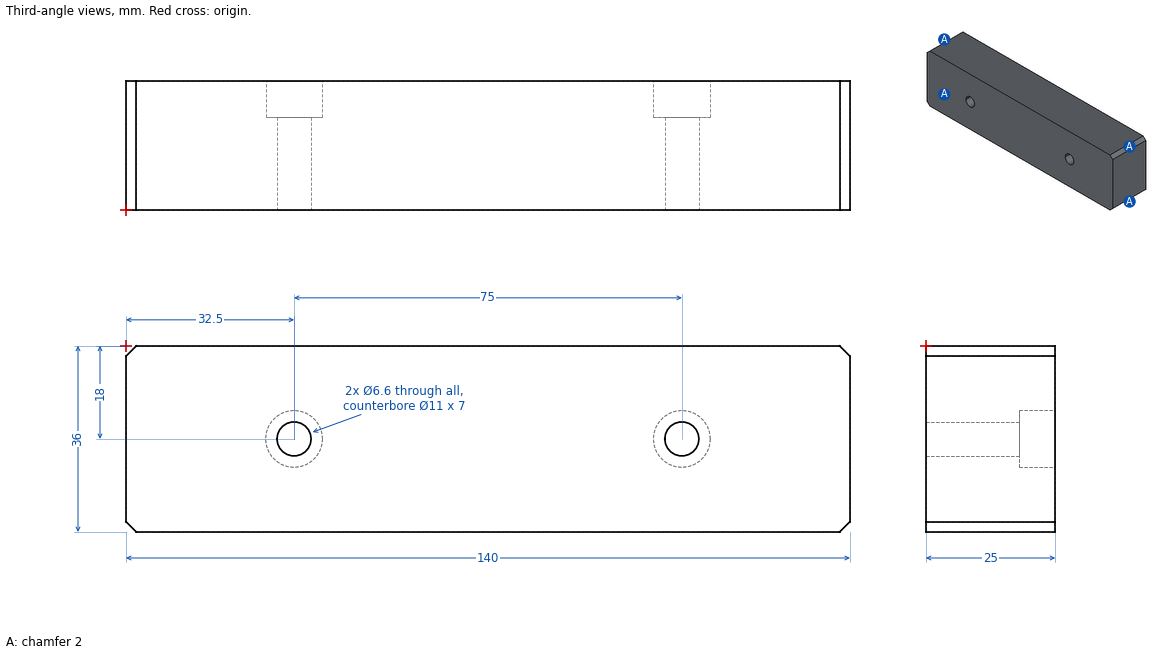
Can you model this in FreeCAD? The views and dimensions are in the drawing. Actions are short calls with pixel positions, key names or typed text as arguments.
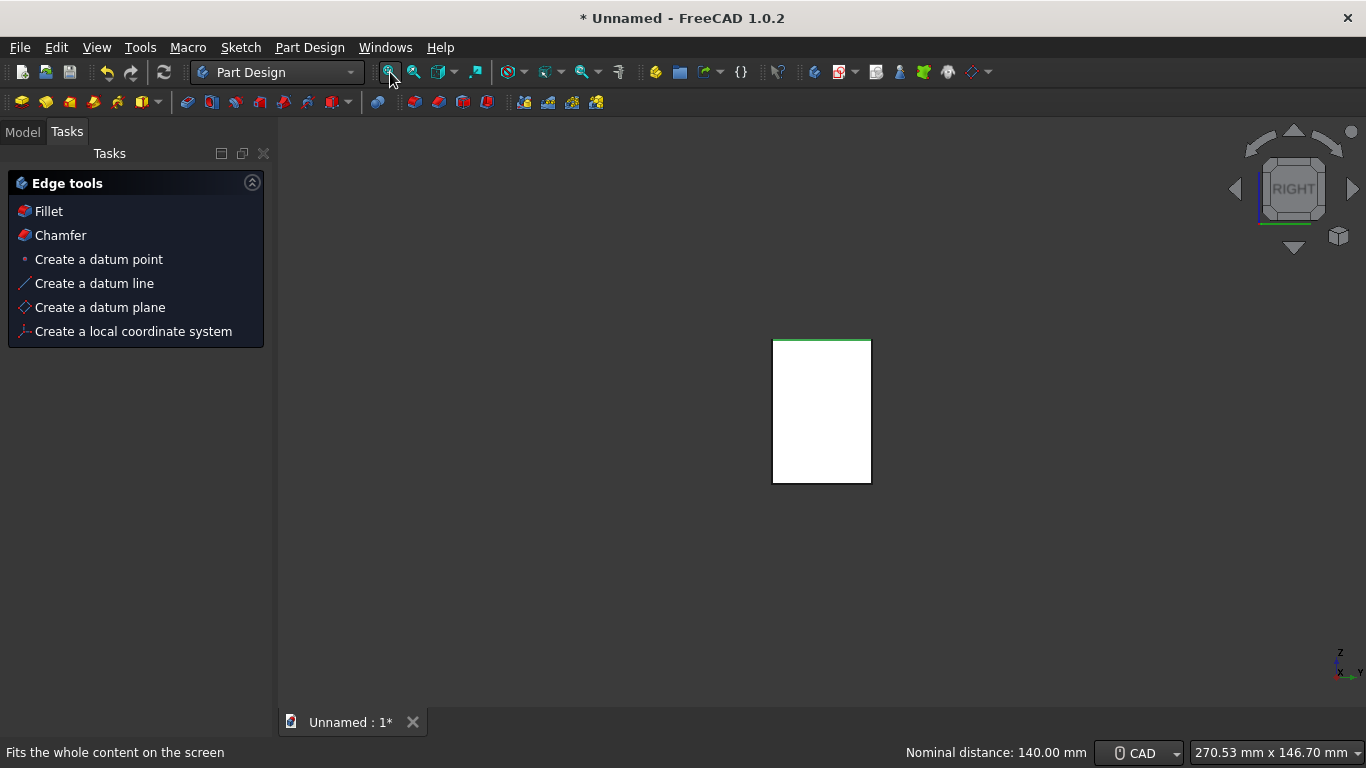
click(822, 483, ctrl)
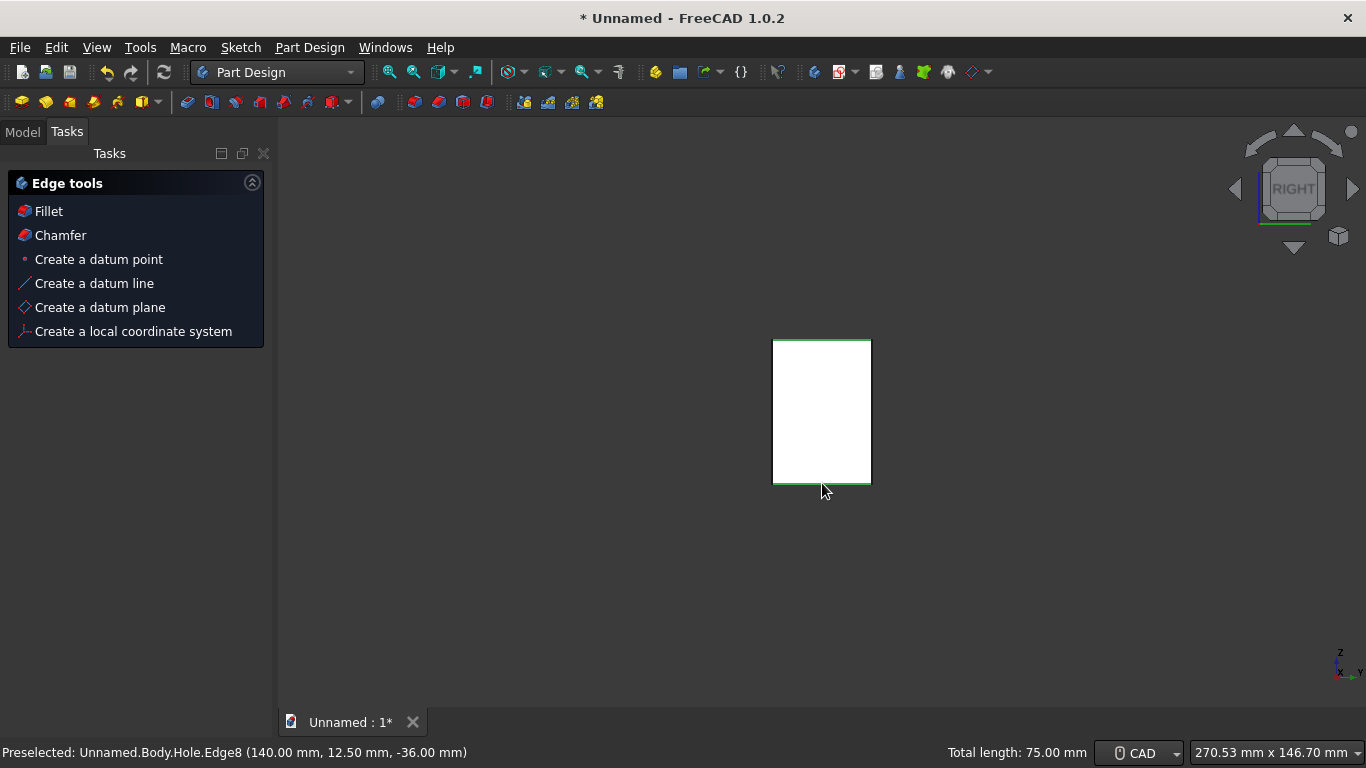
key(5)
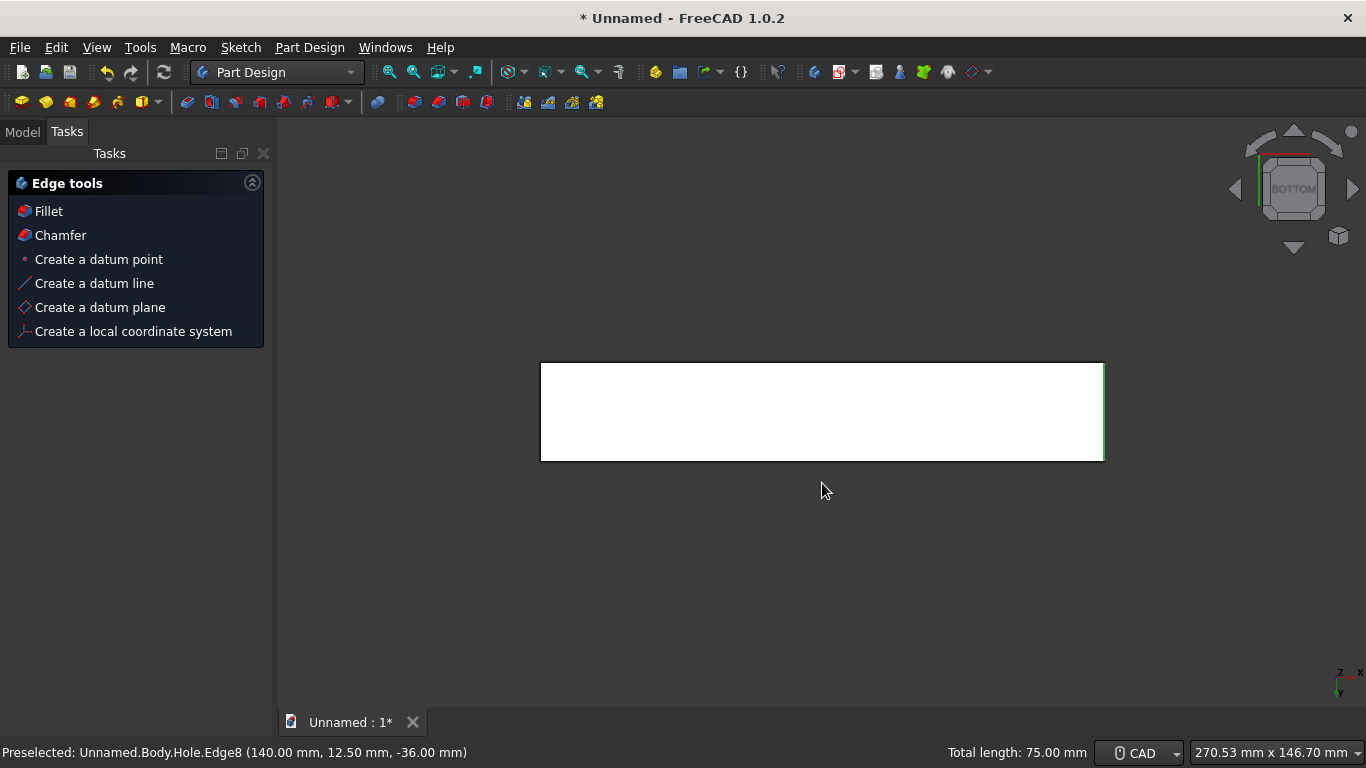
click(540, 411, ctrl)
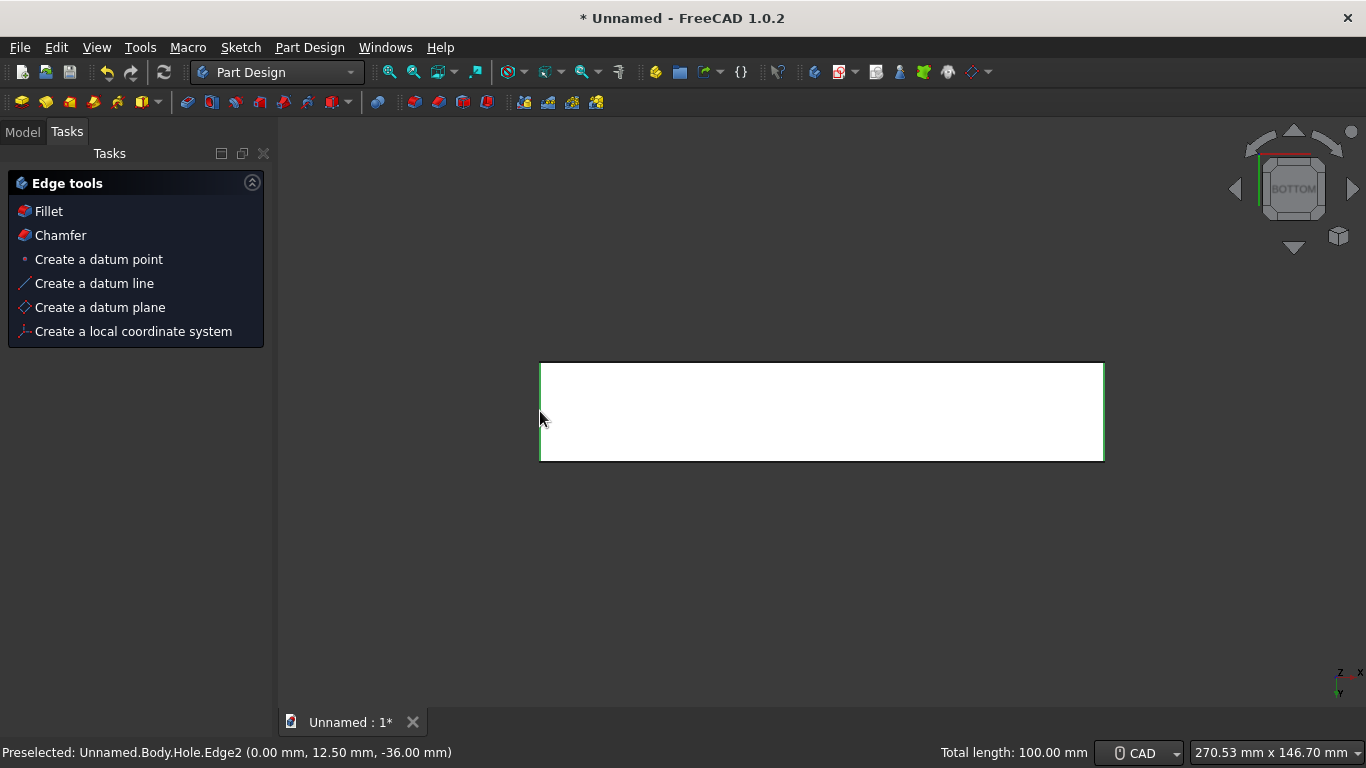
click(440, 102)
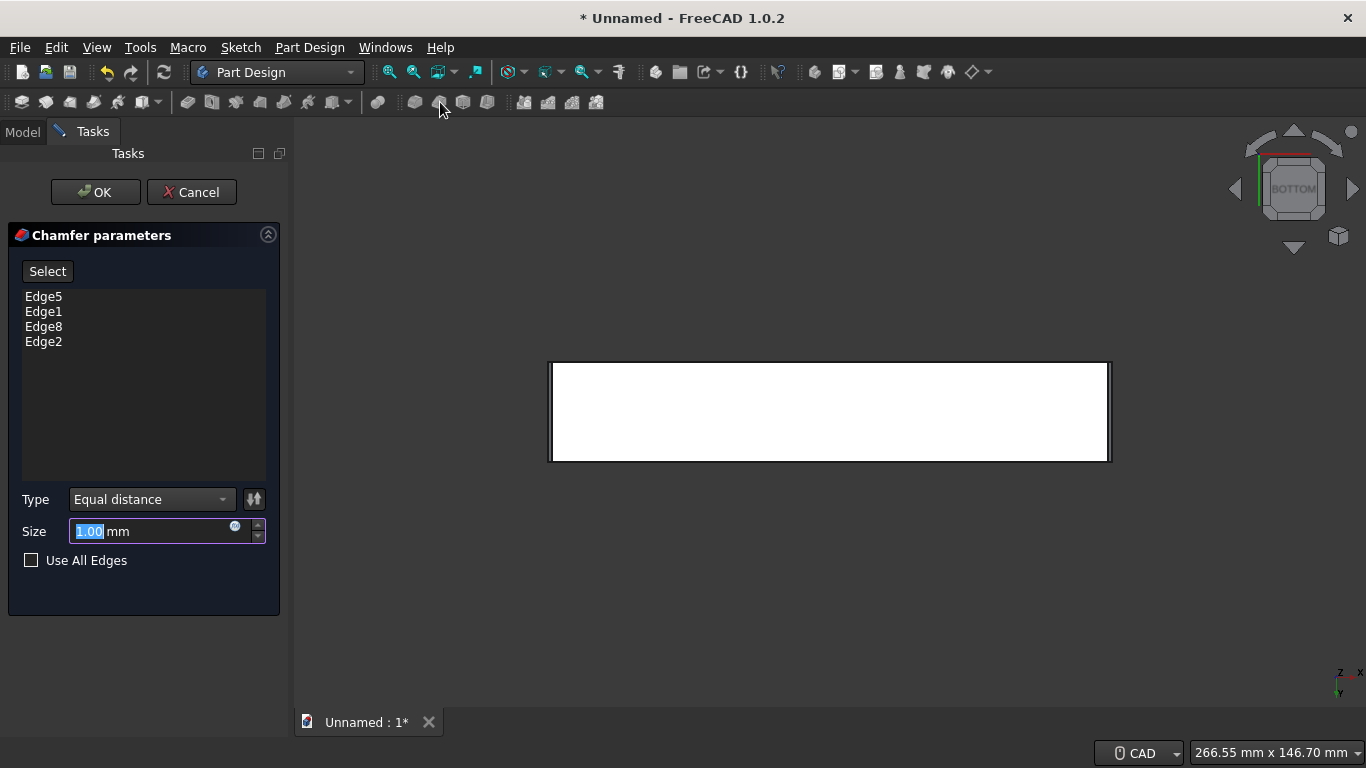
text(2)
key(Tab)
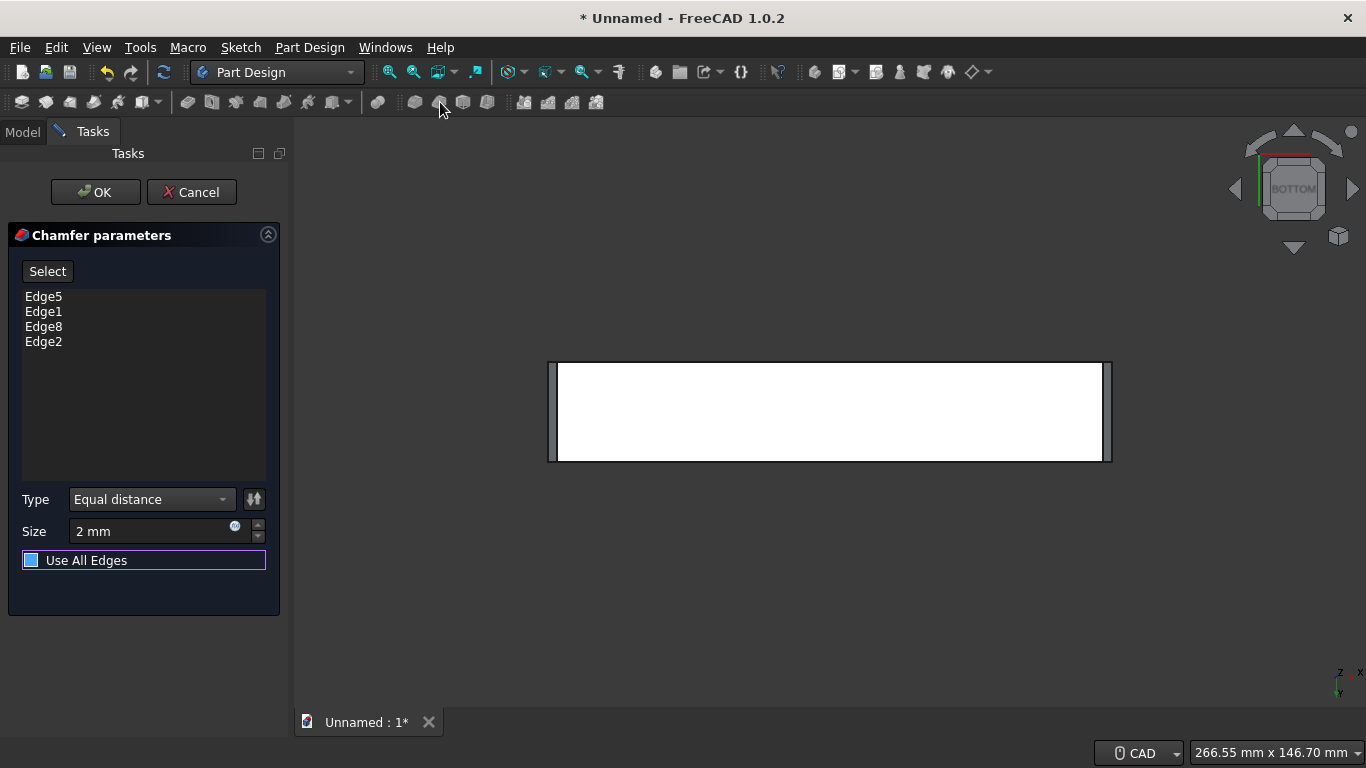
click(96, 192)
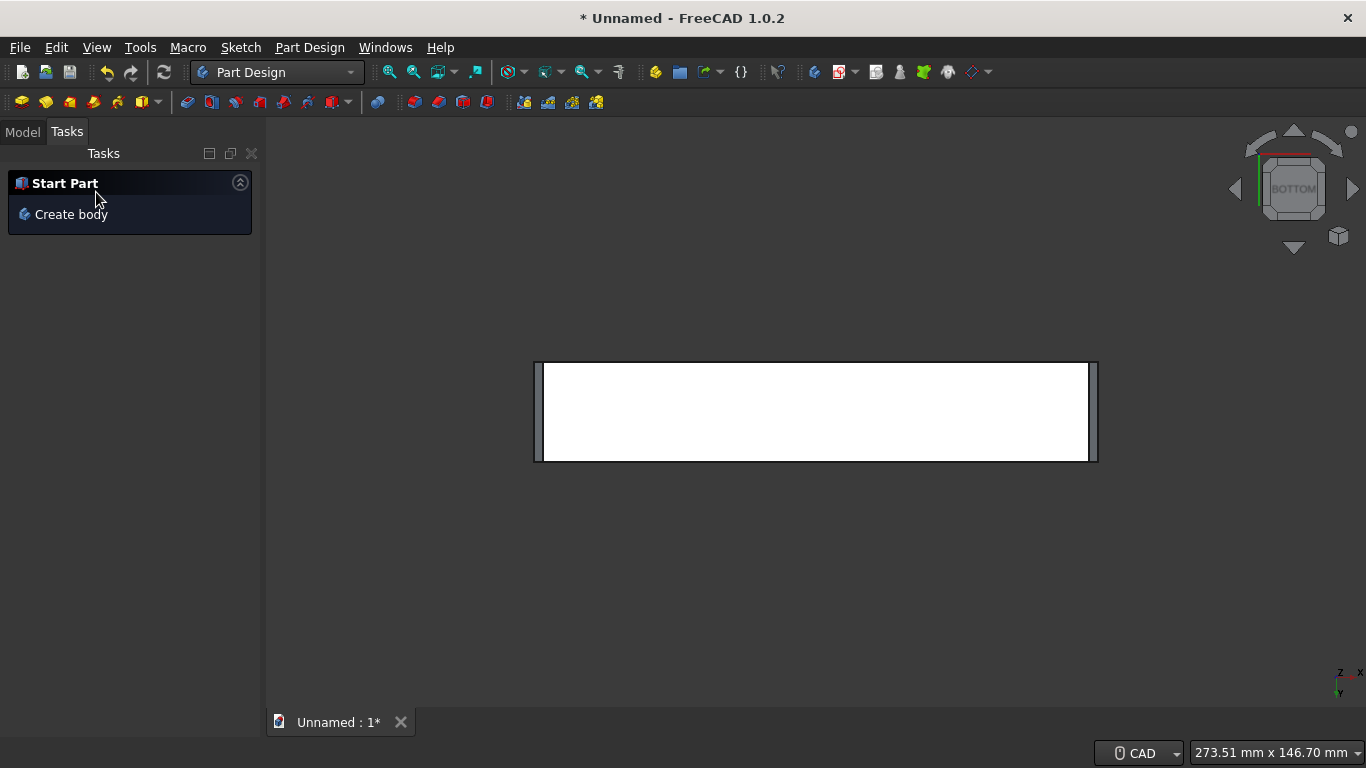
key(0)